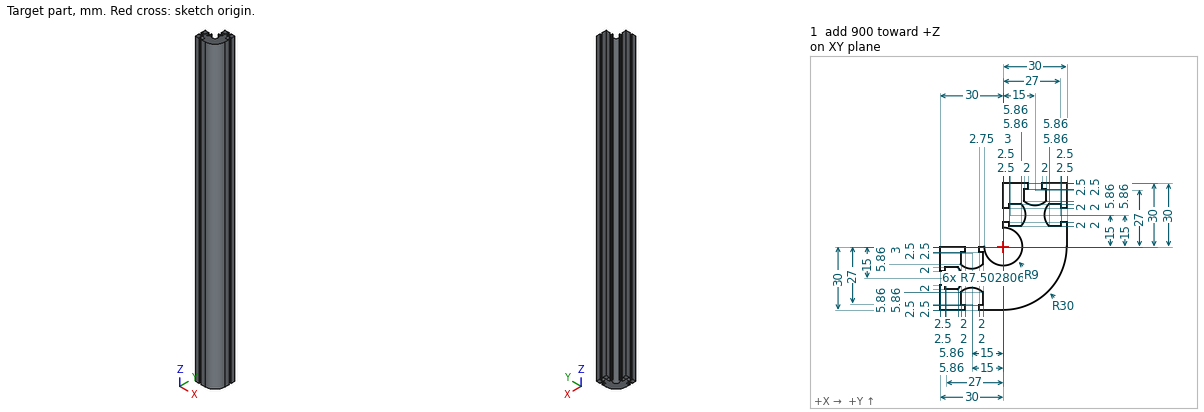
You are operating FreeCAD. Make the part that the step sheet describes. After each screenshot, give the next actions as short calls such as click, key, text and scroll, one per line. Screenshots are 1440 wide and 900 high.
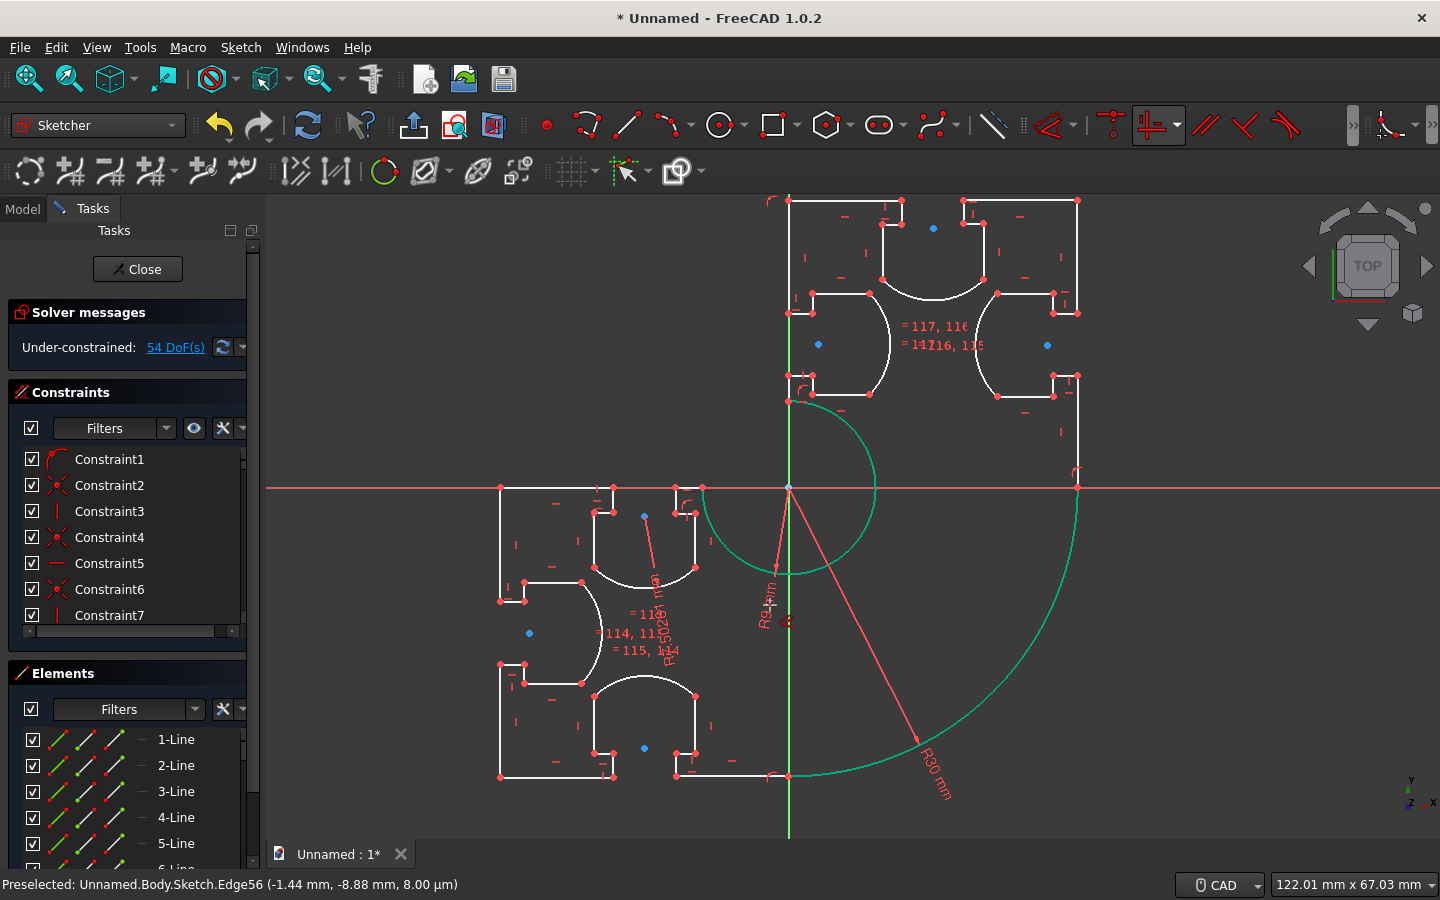
scroll(685, 514, up, 4)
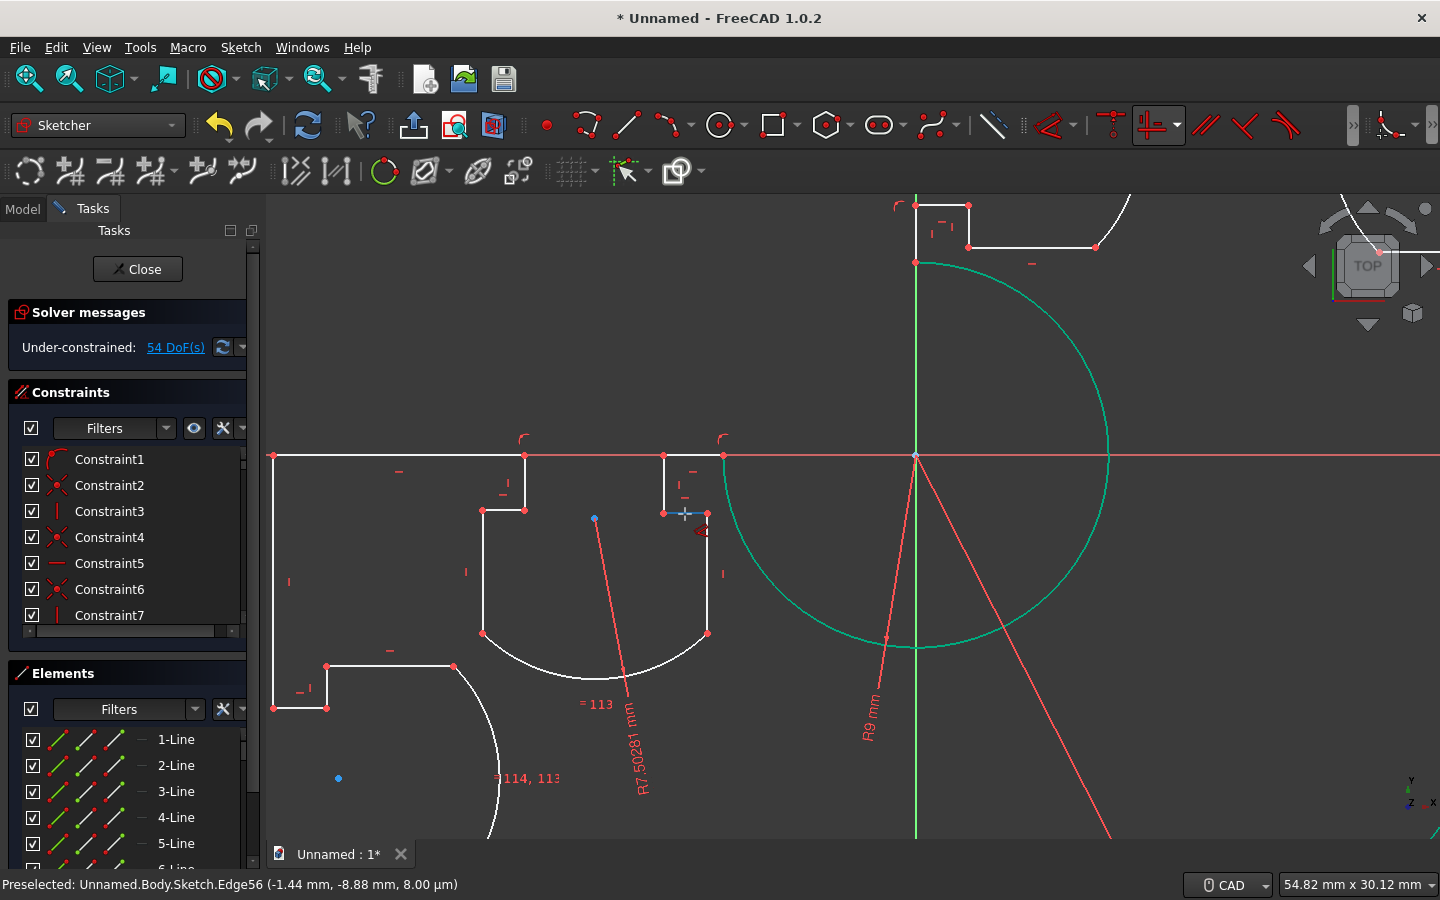
click(685, 513)
click(685, 547)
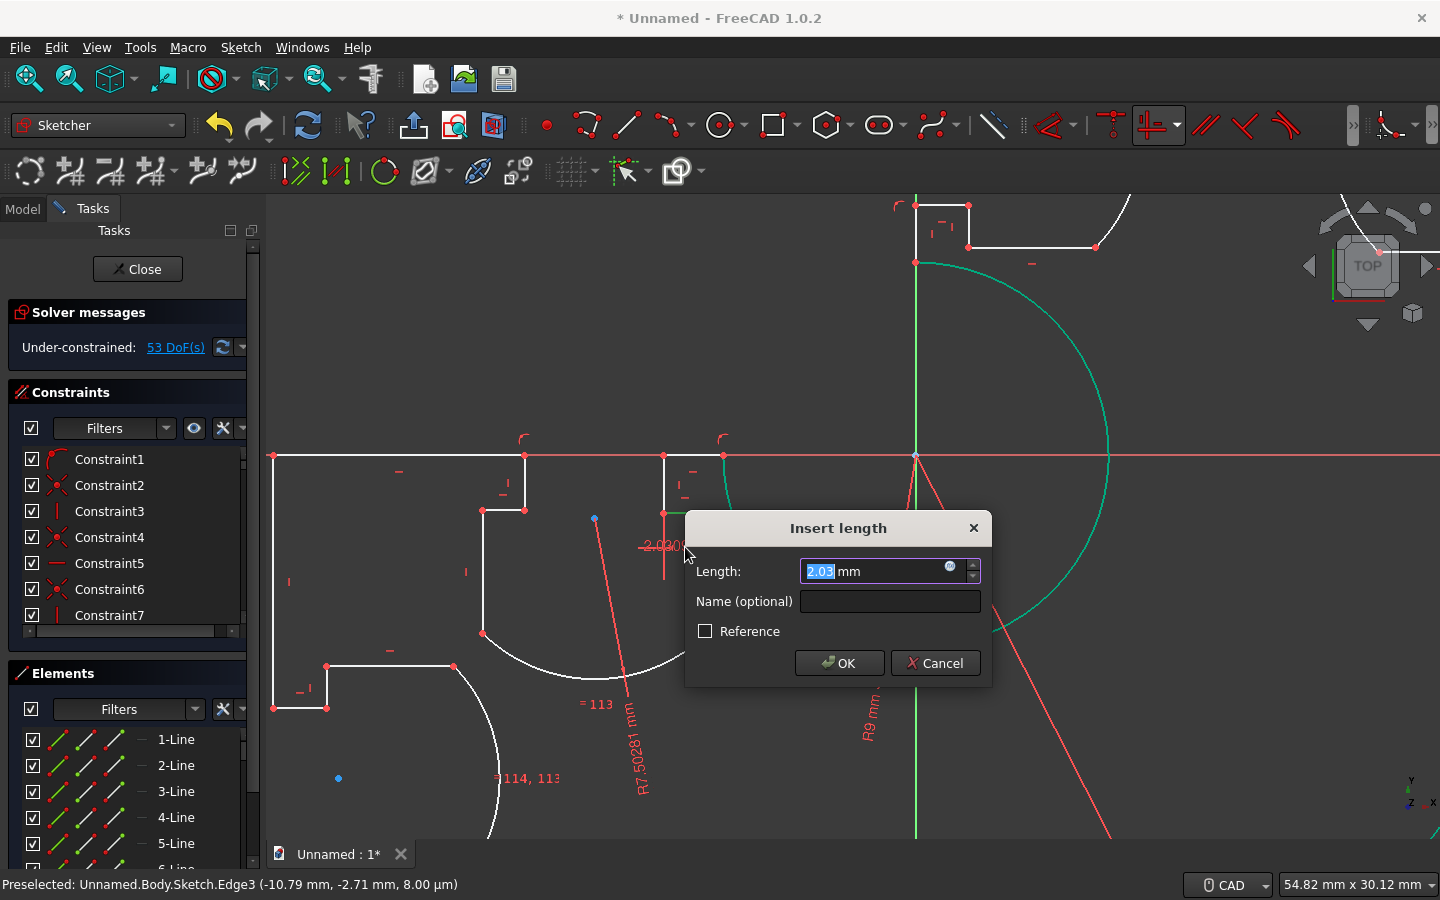
text(2)
key(Return)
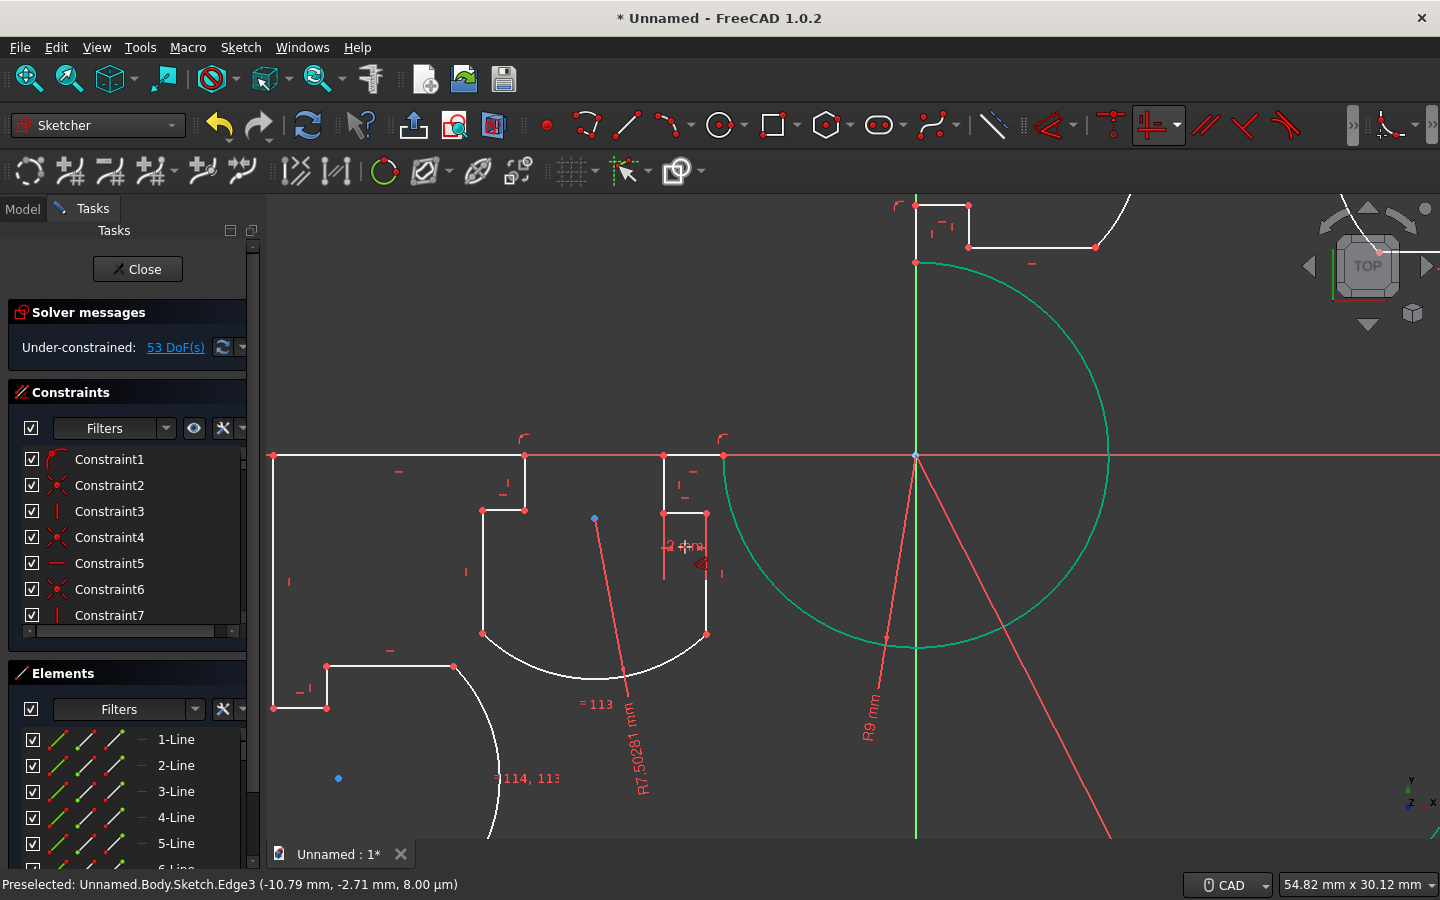
click(495, 510)
click(504, 544)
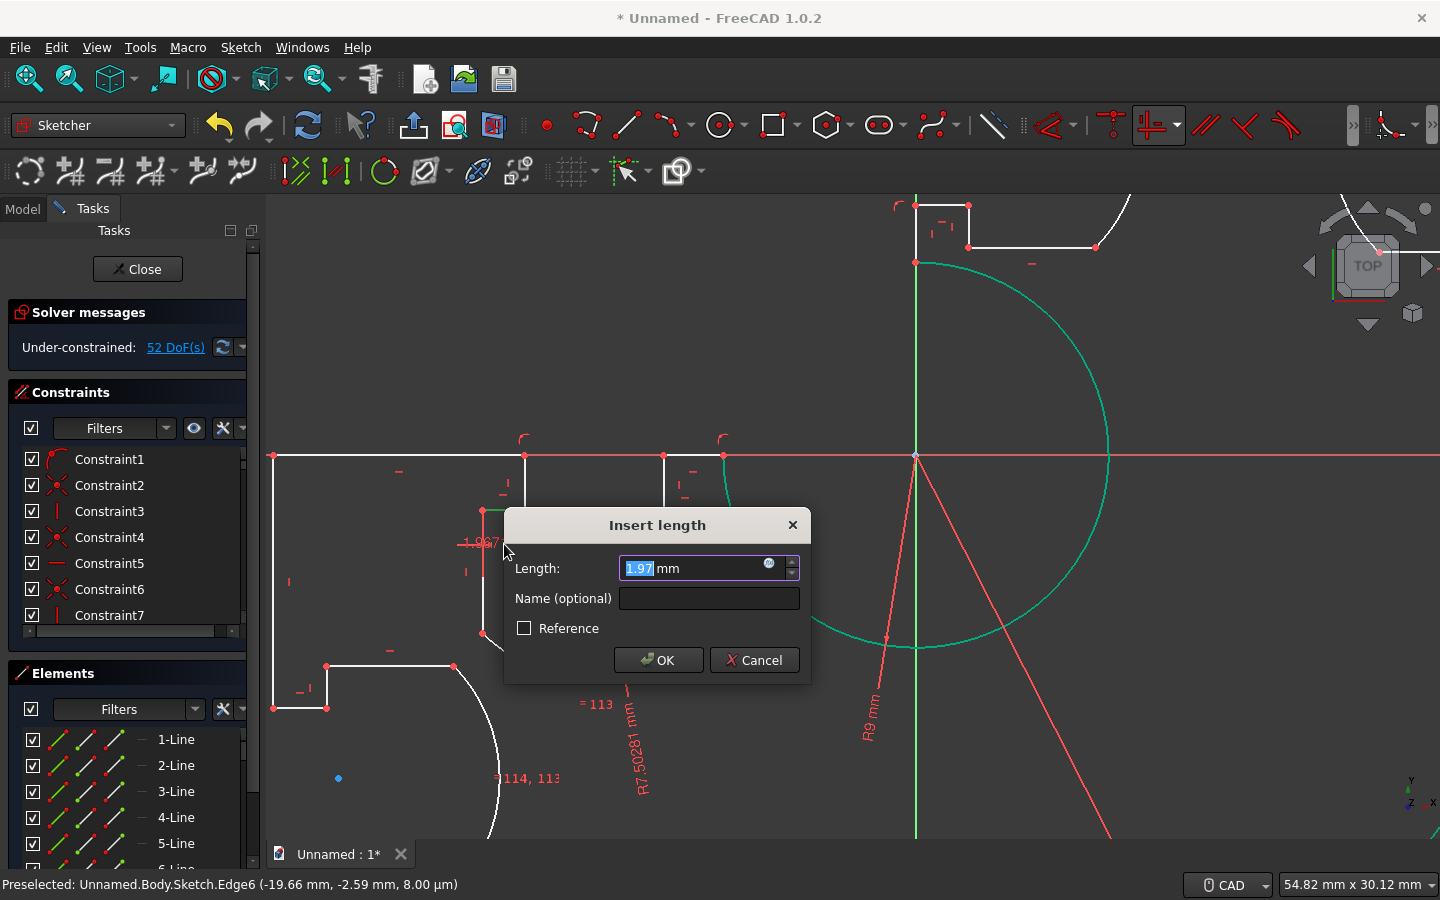
text(2)
key(Return)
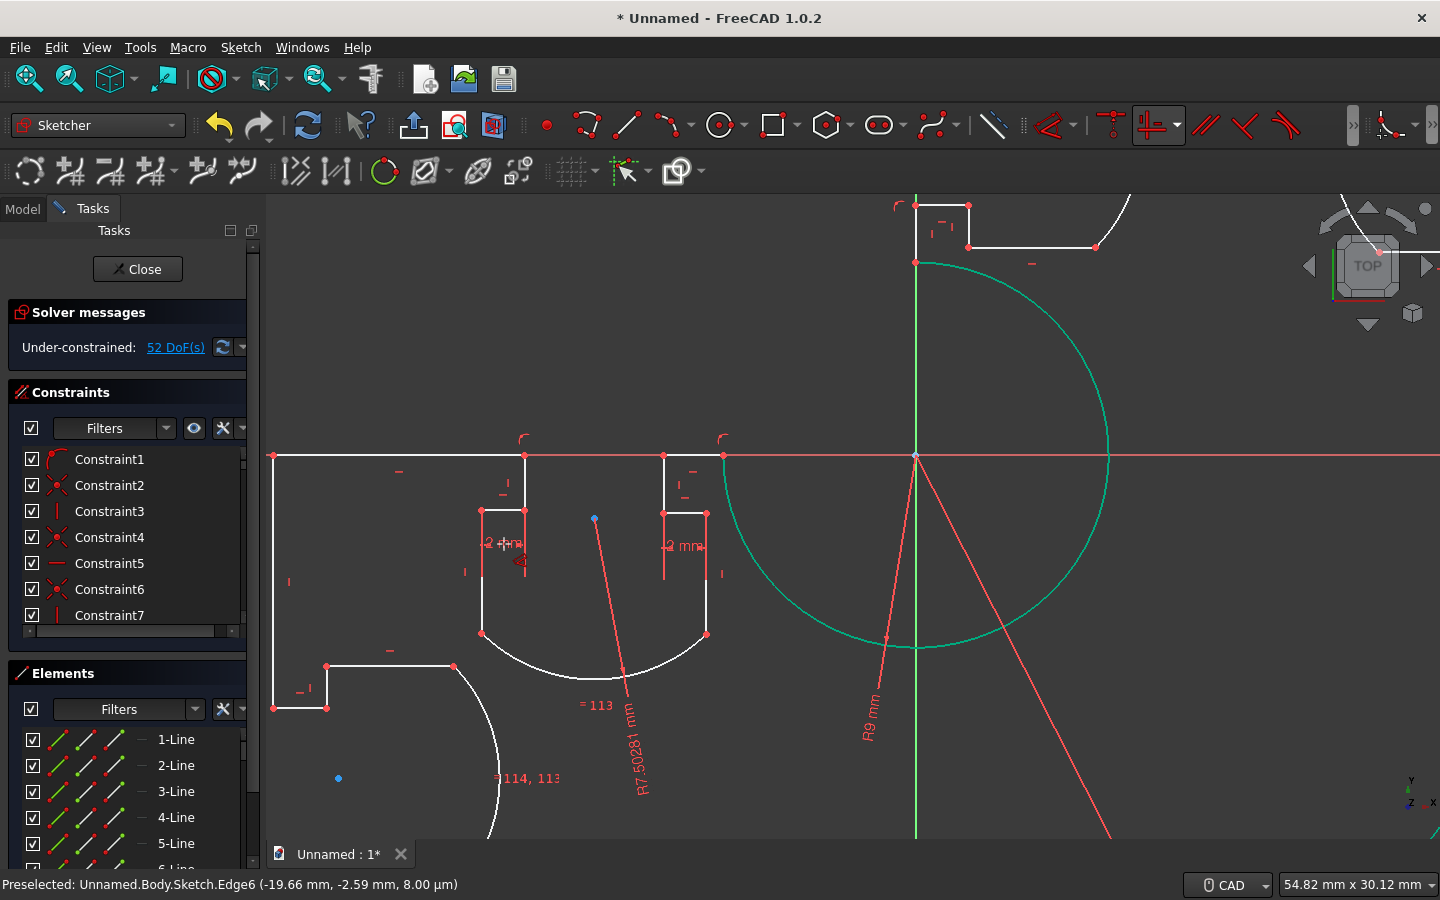
click(327, 696)
click(361, 687)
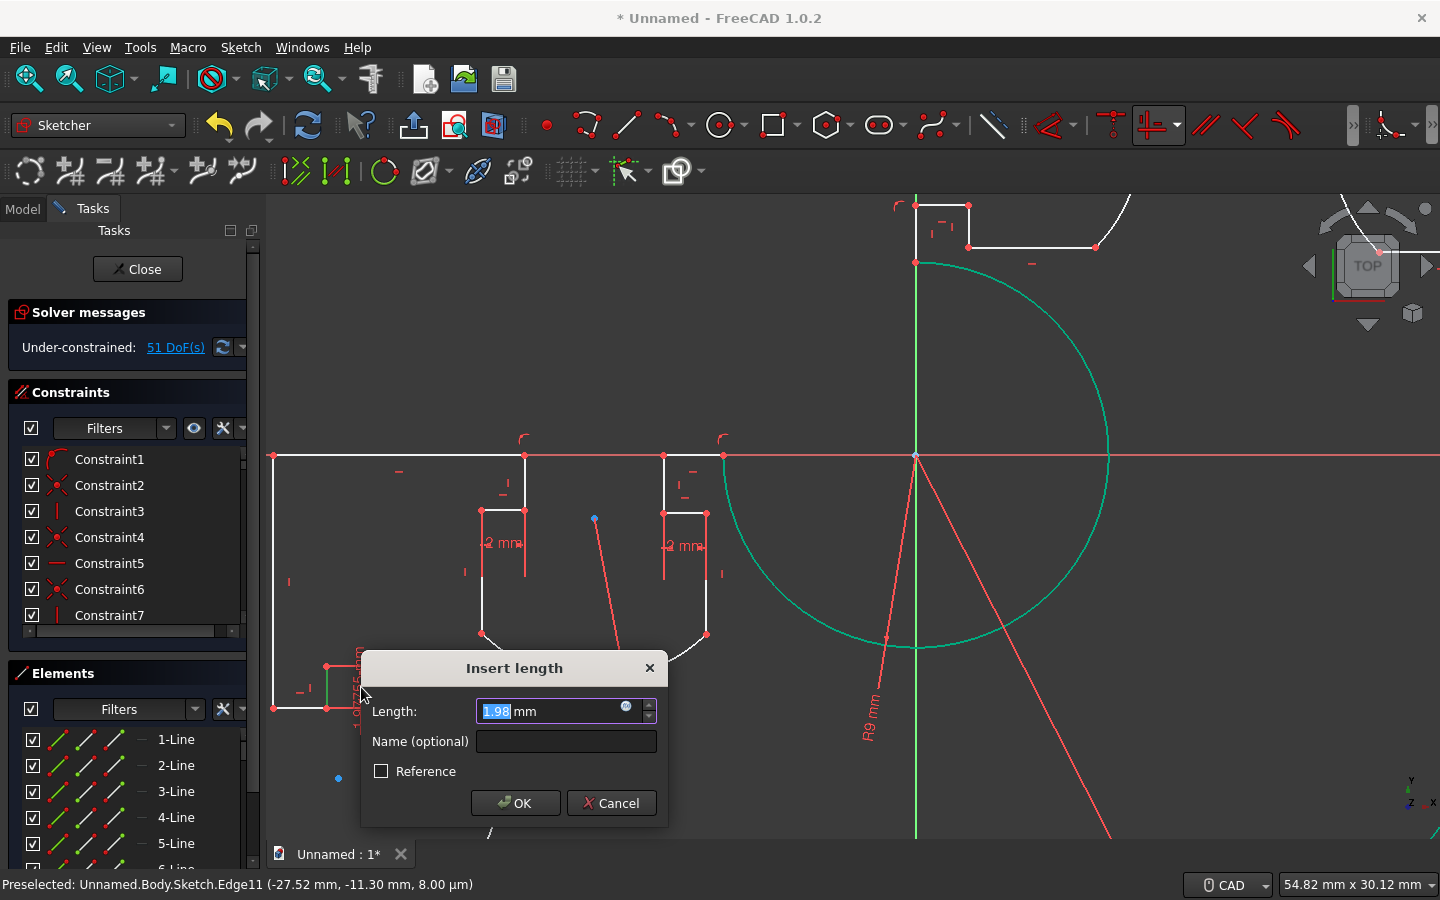
text(2)
key(Return)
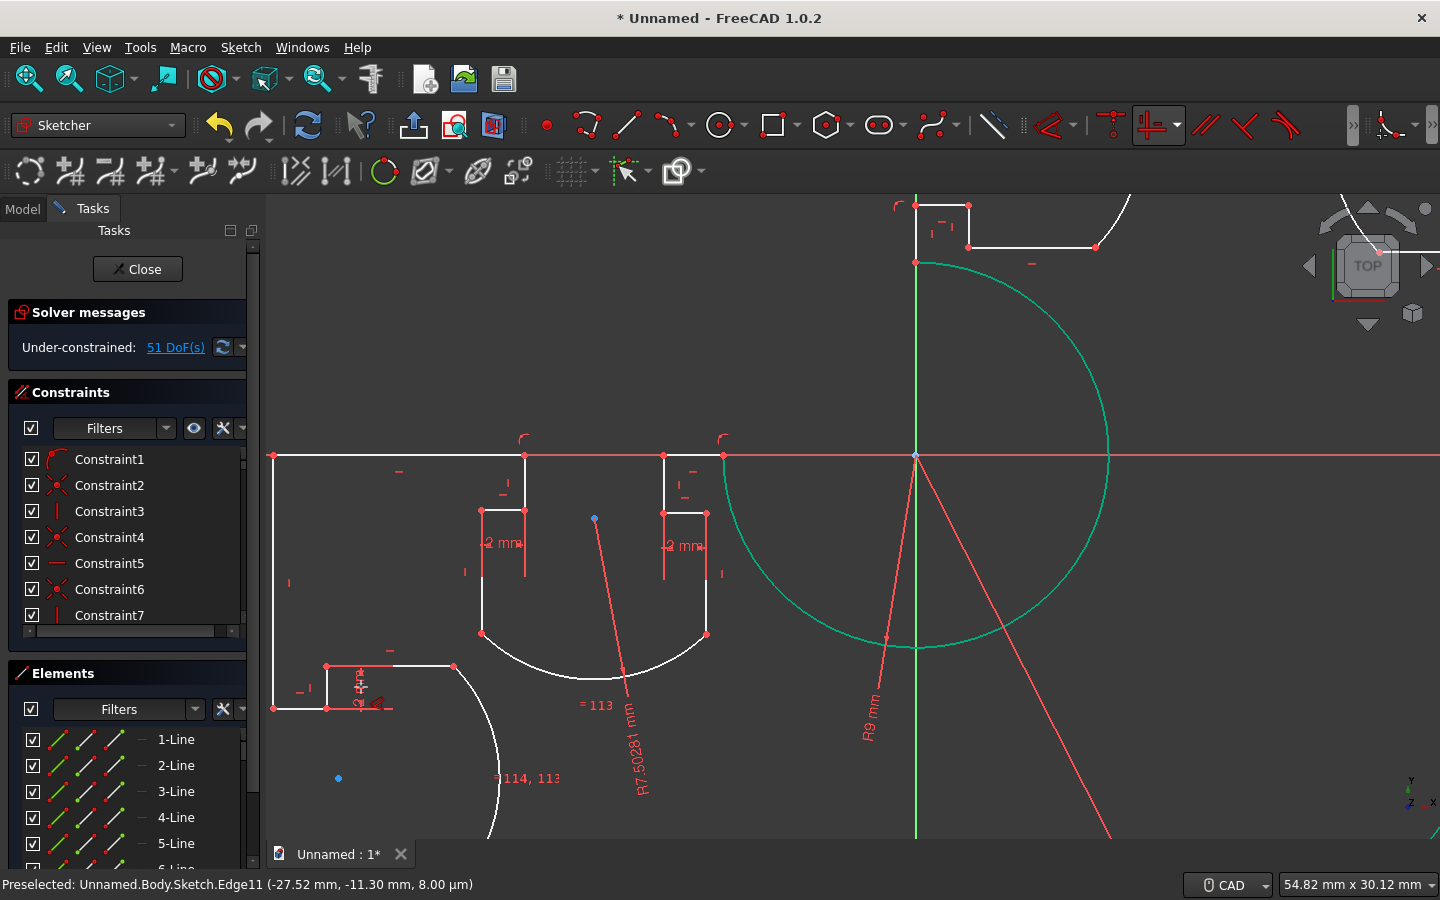
scroll(728, 543, down, 6)